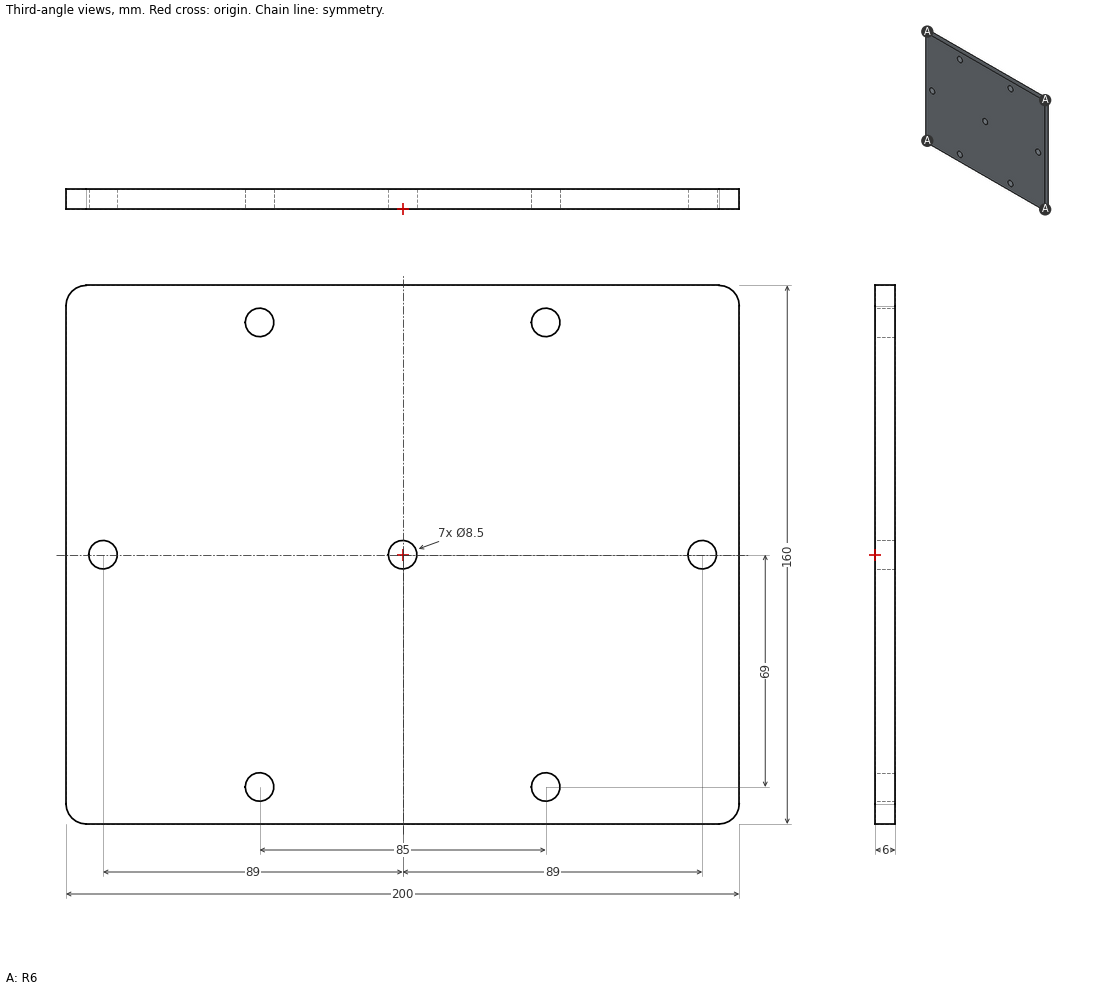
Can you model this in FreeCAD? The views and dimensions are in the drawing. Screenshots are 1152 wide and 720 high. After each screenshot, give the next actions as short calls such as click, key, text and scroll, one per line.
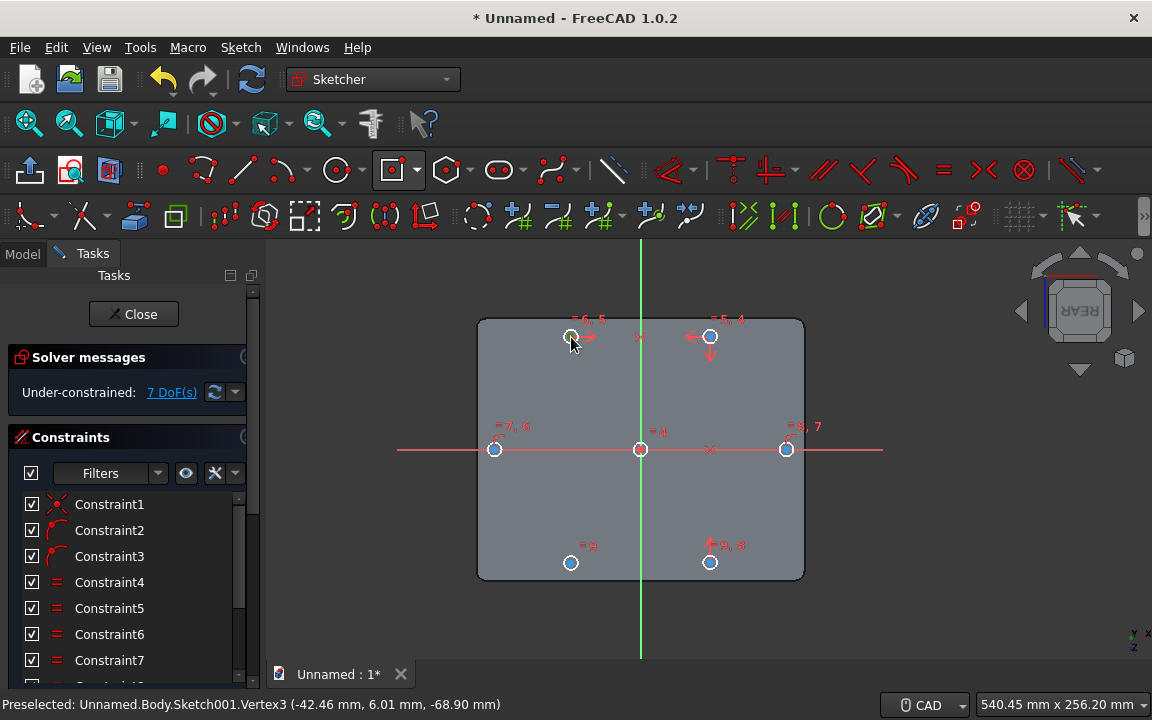
click(571, 563)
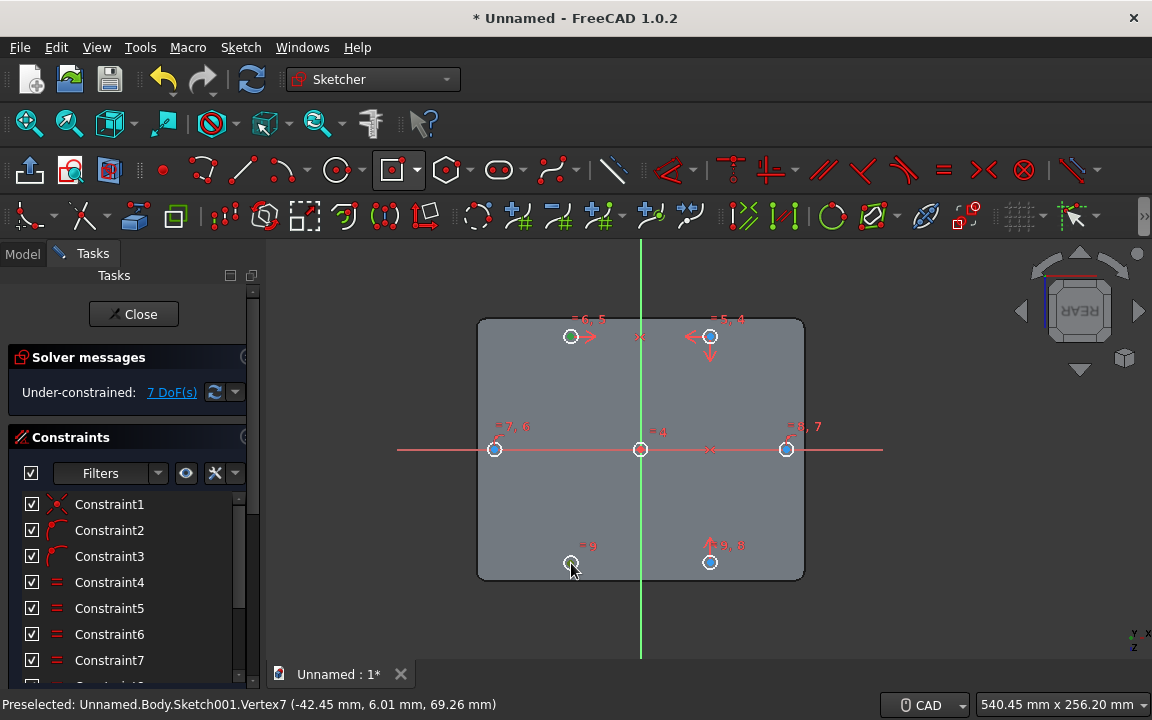
click(393, 450)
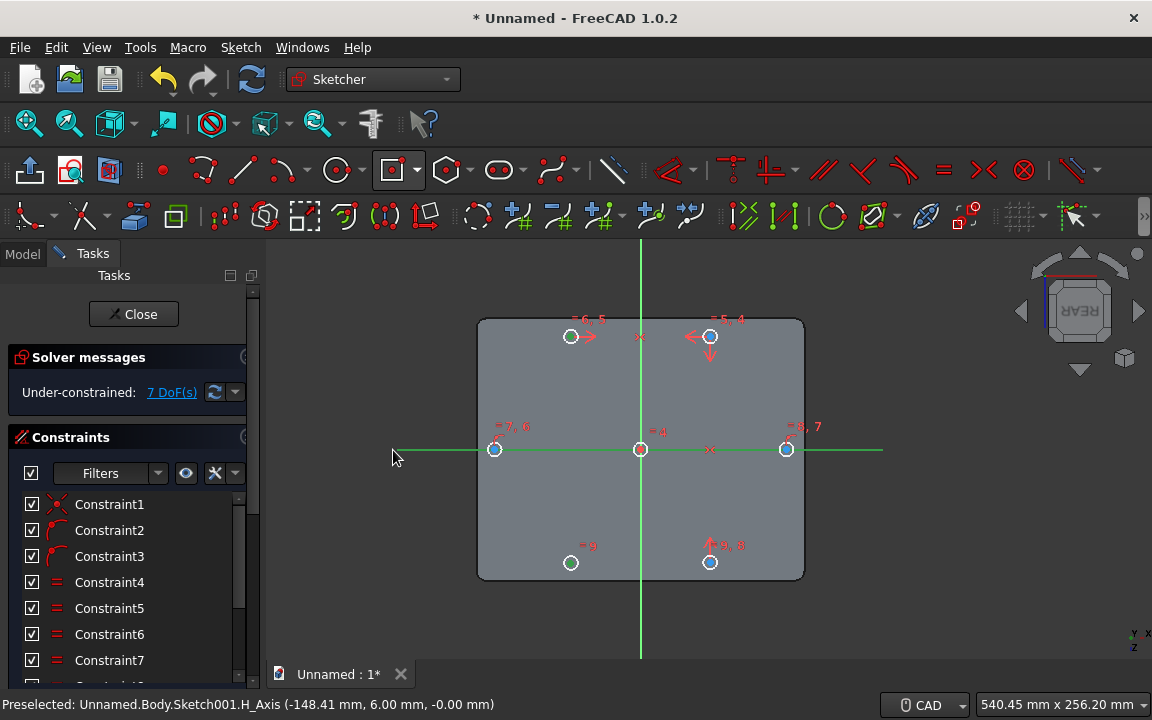
click(984, 170)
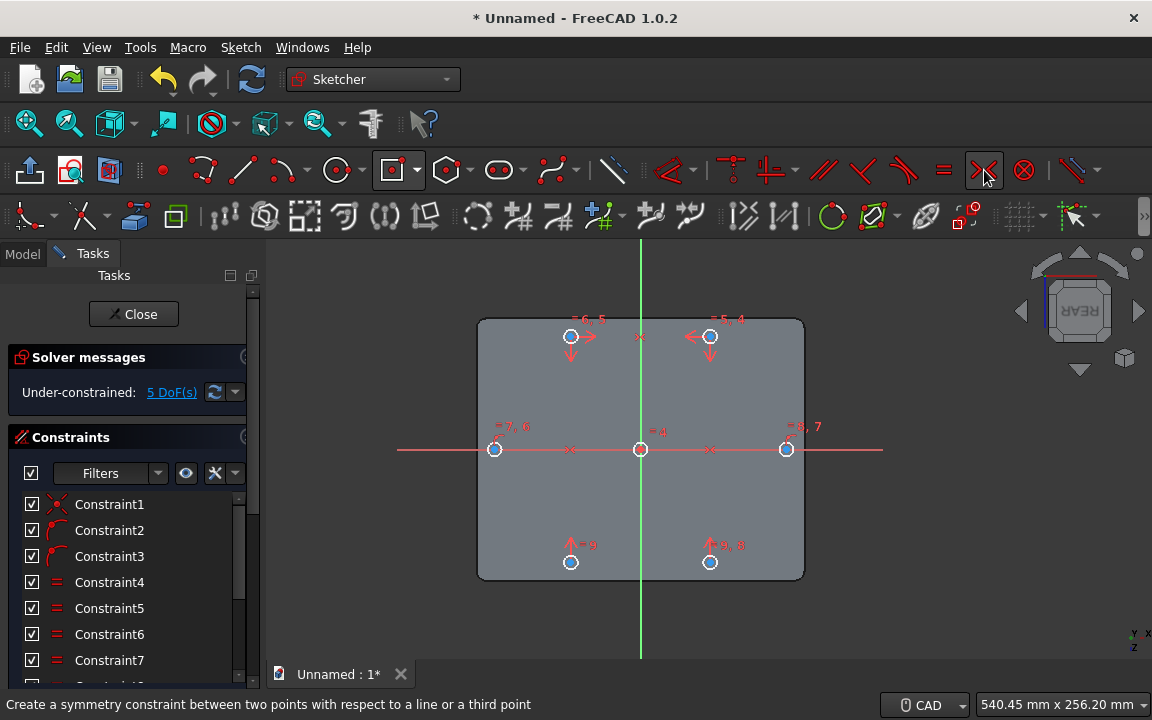
click(668, 170)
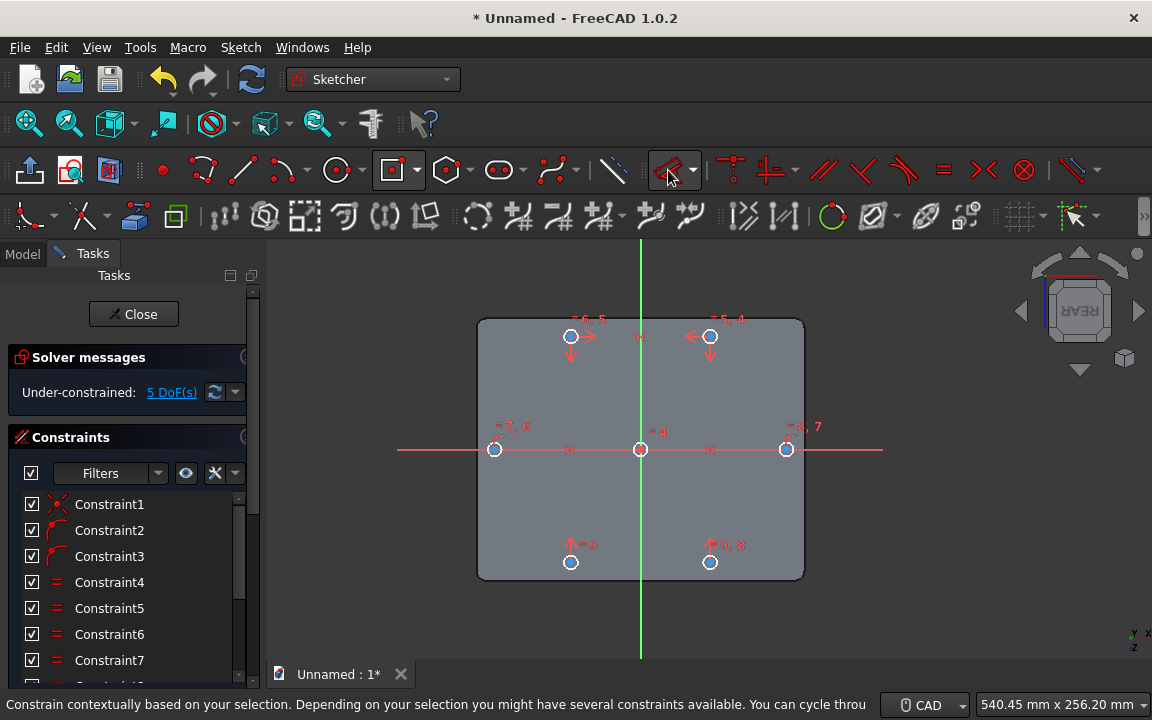
scroll(641, 443, up, 6)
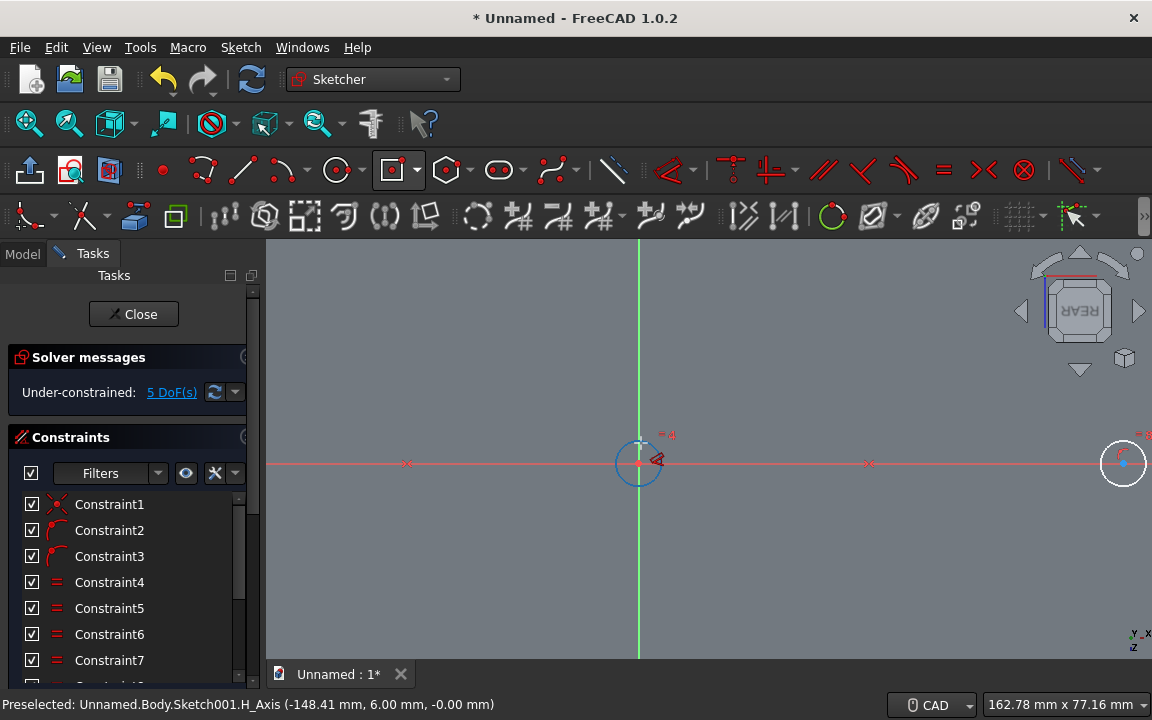
click(639, 441)
click(666, 416)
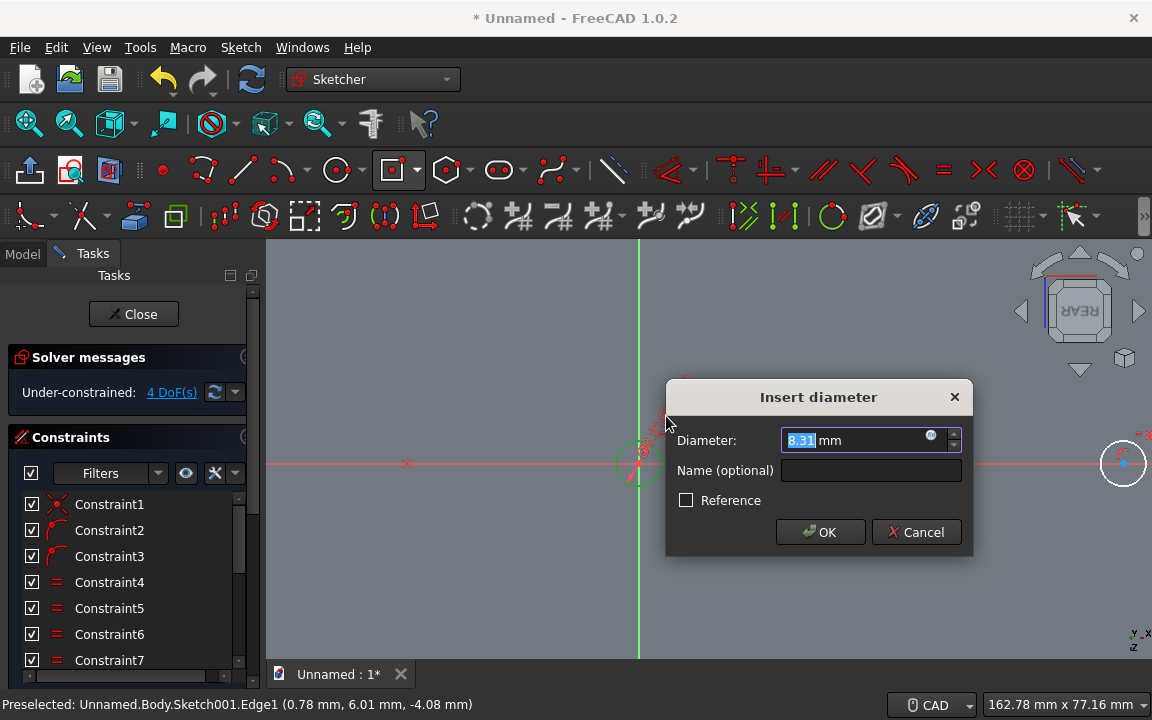
text(8.5)
key(Return)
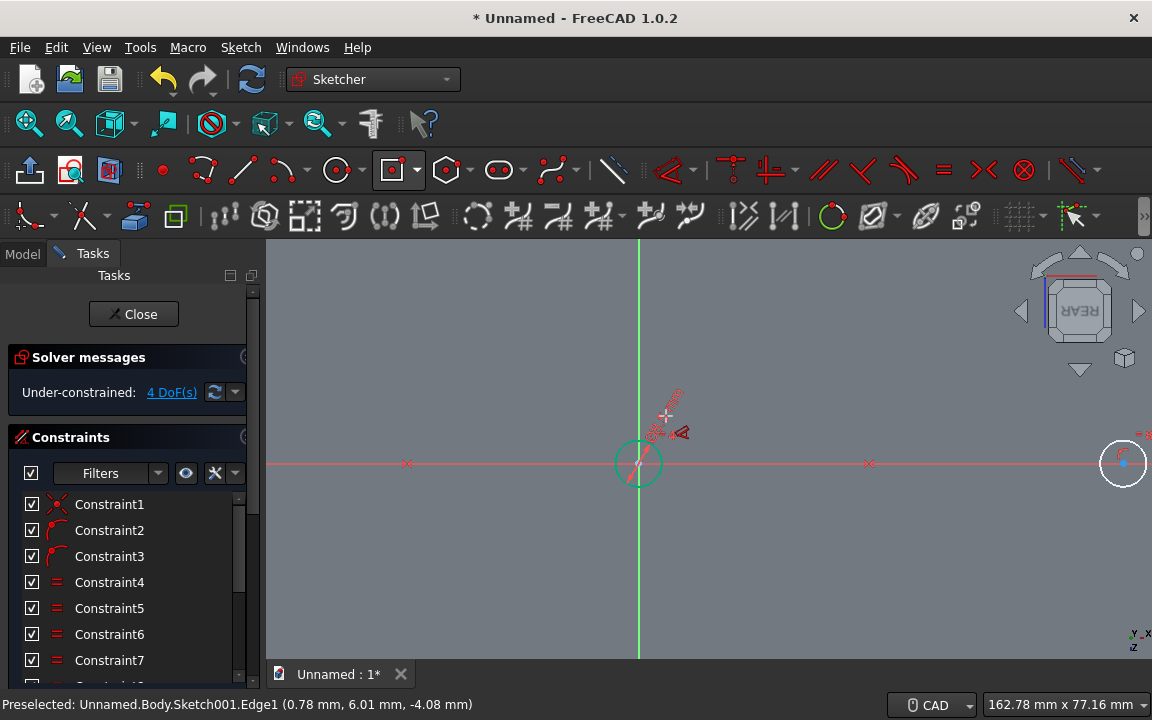
scroll(641, 443, down, 6)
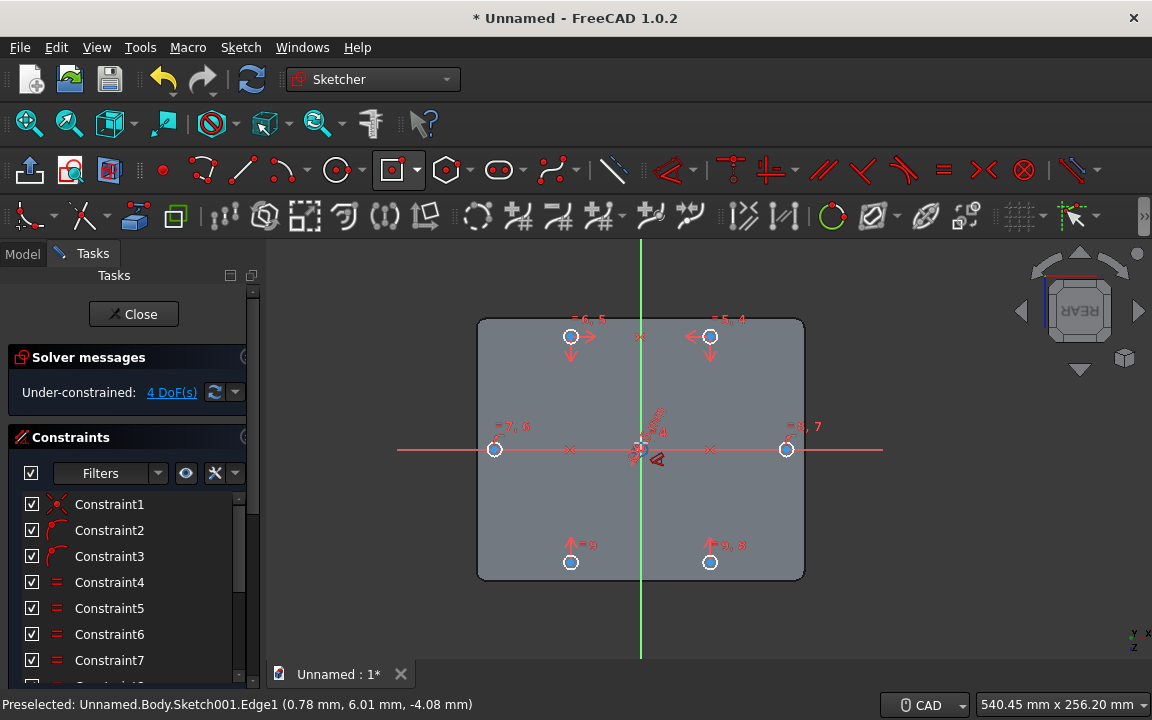
click(710, 337)
click(744, 393)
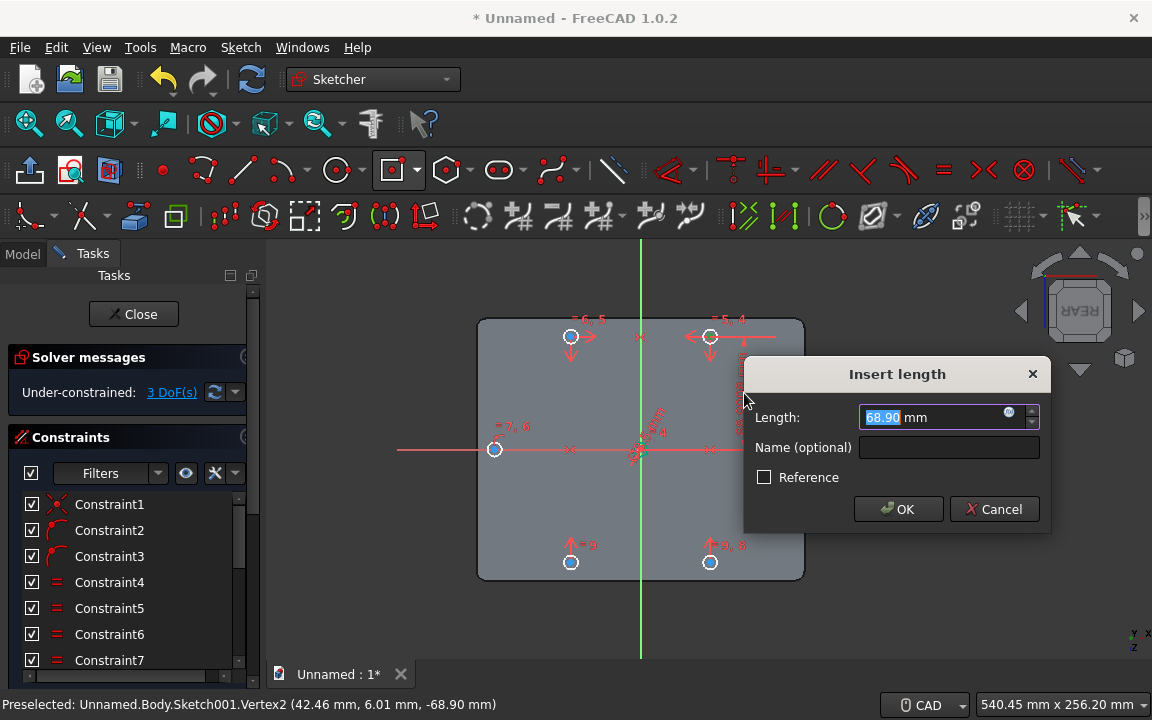
text(69)
key(Return)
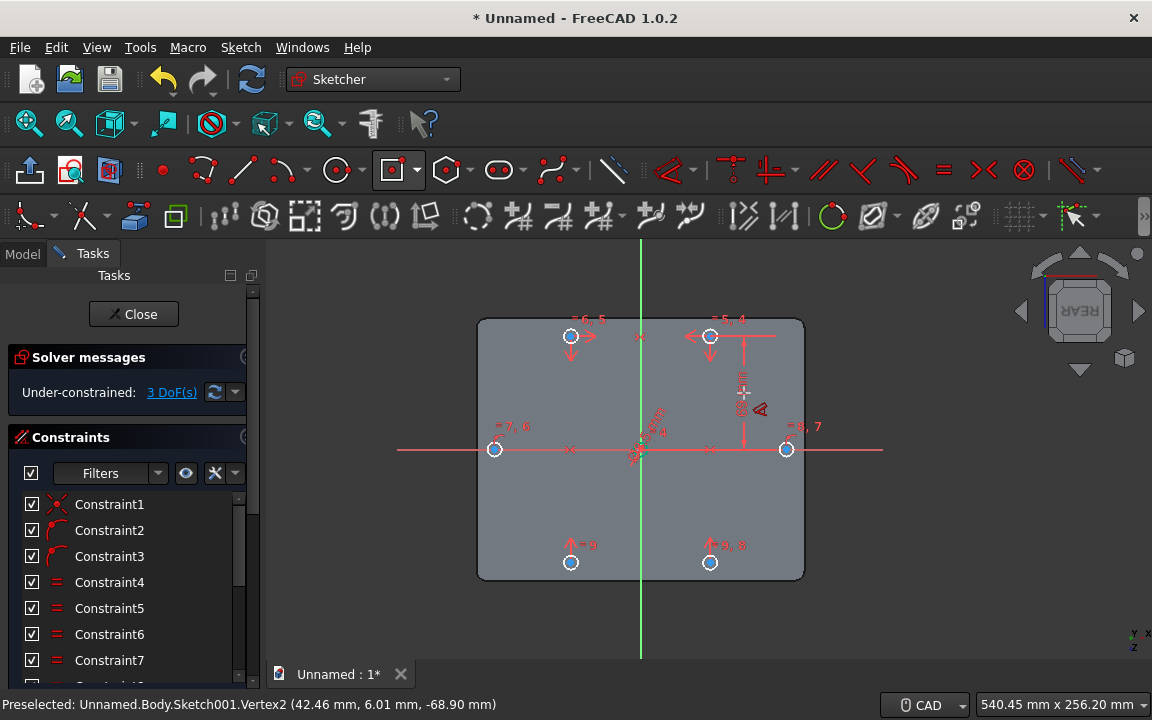
click(495, 450)
click(568, 484)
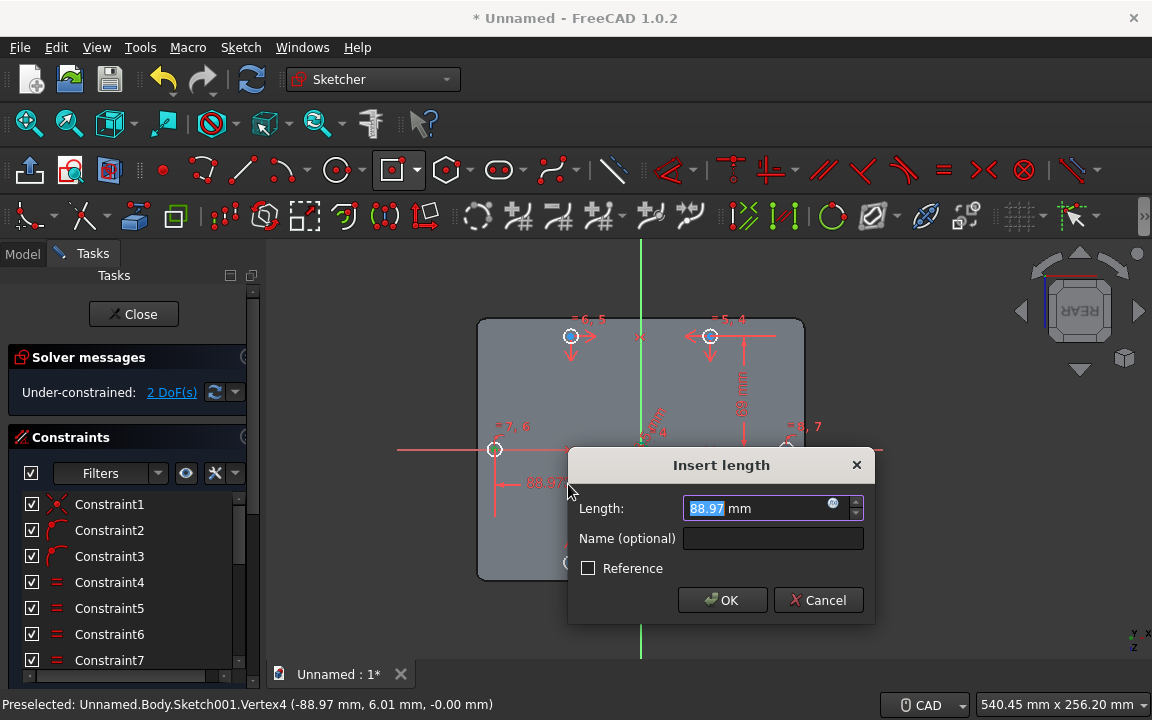
text(89)
key(Return)